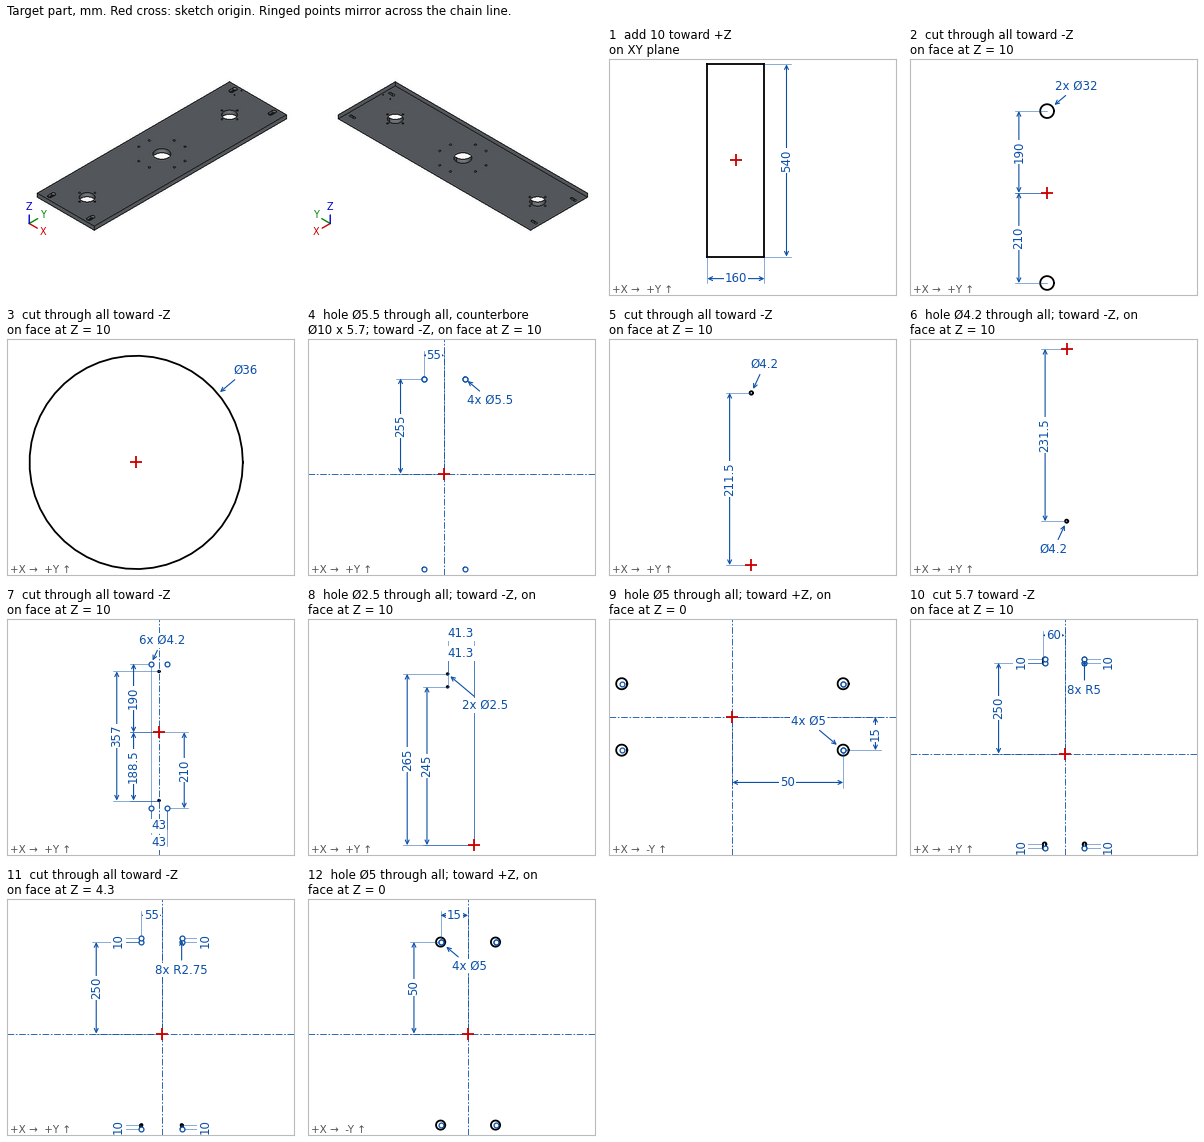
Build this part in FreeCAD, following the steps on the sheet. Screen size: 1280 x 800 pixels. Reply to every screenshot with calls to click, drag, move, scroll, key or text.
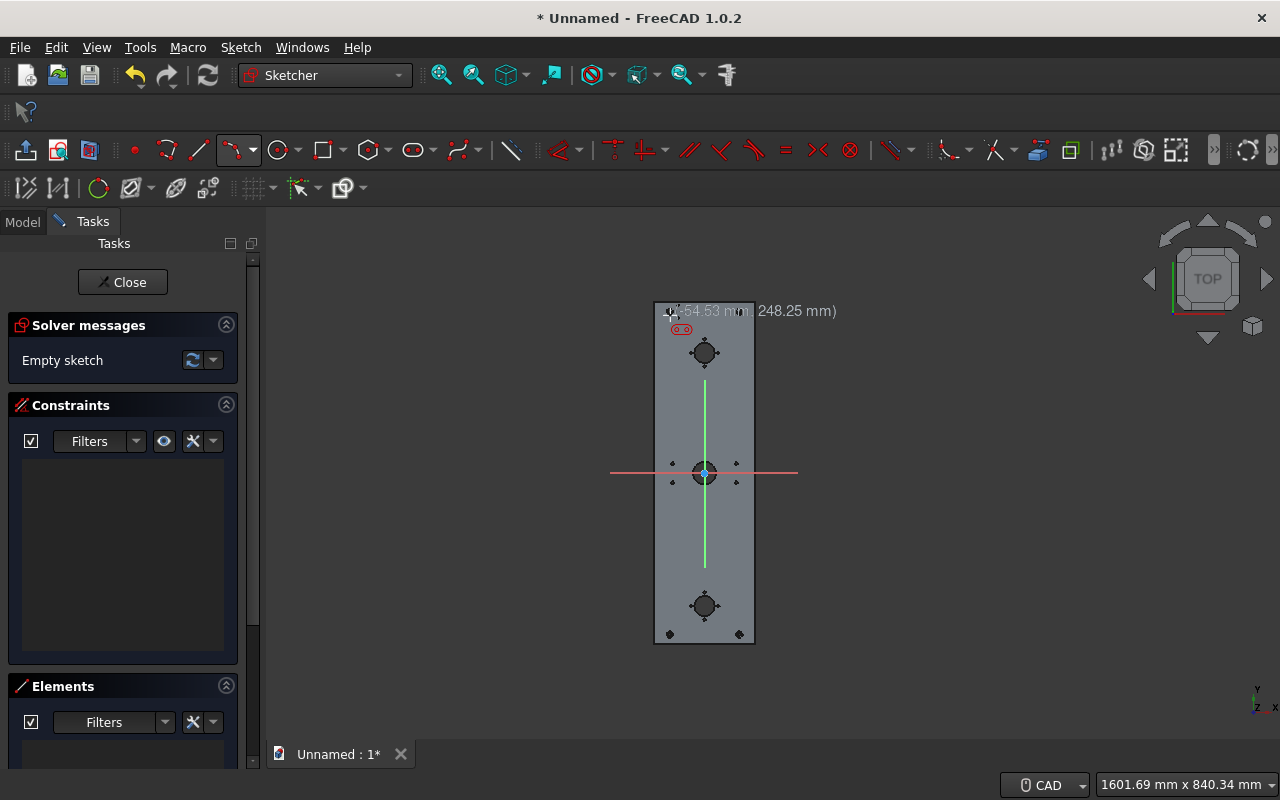
click(670, 315)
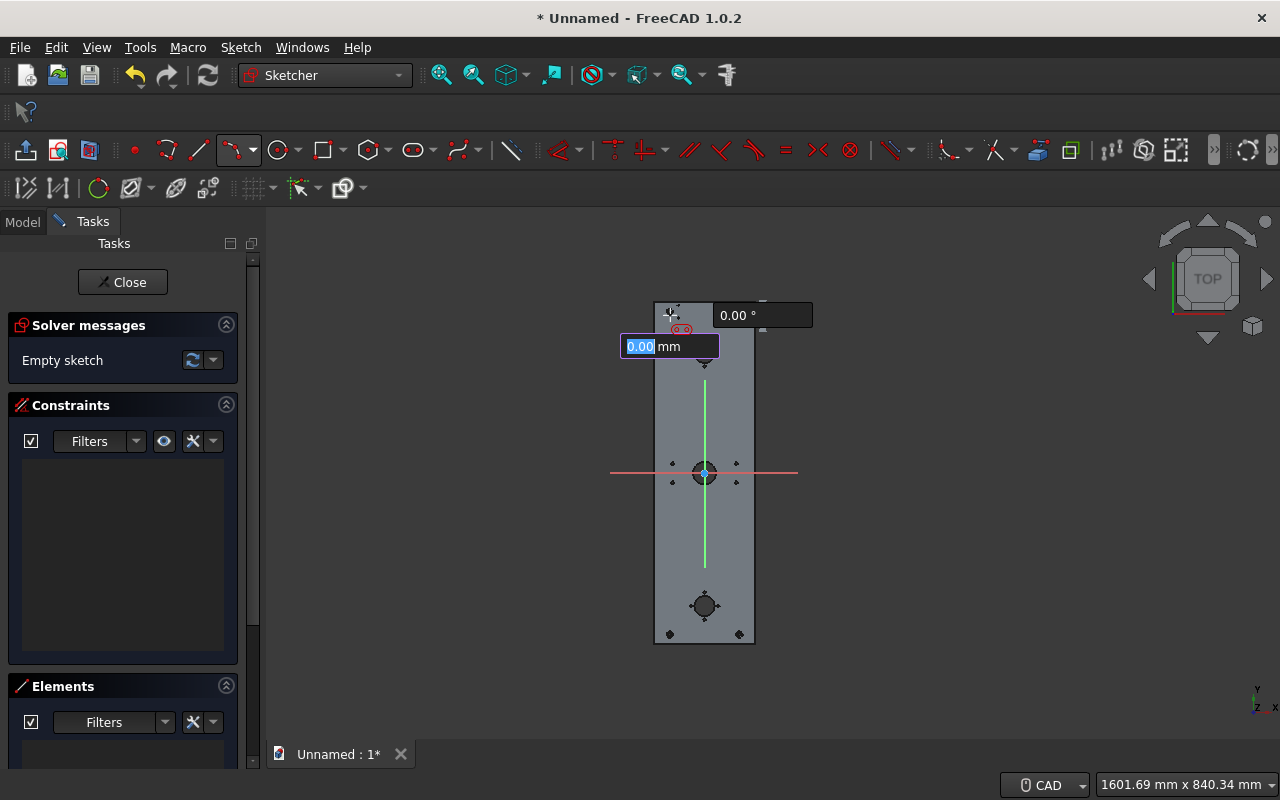
scroll(670, 309, up, 5)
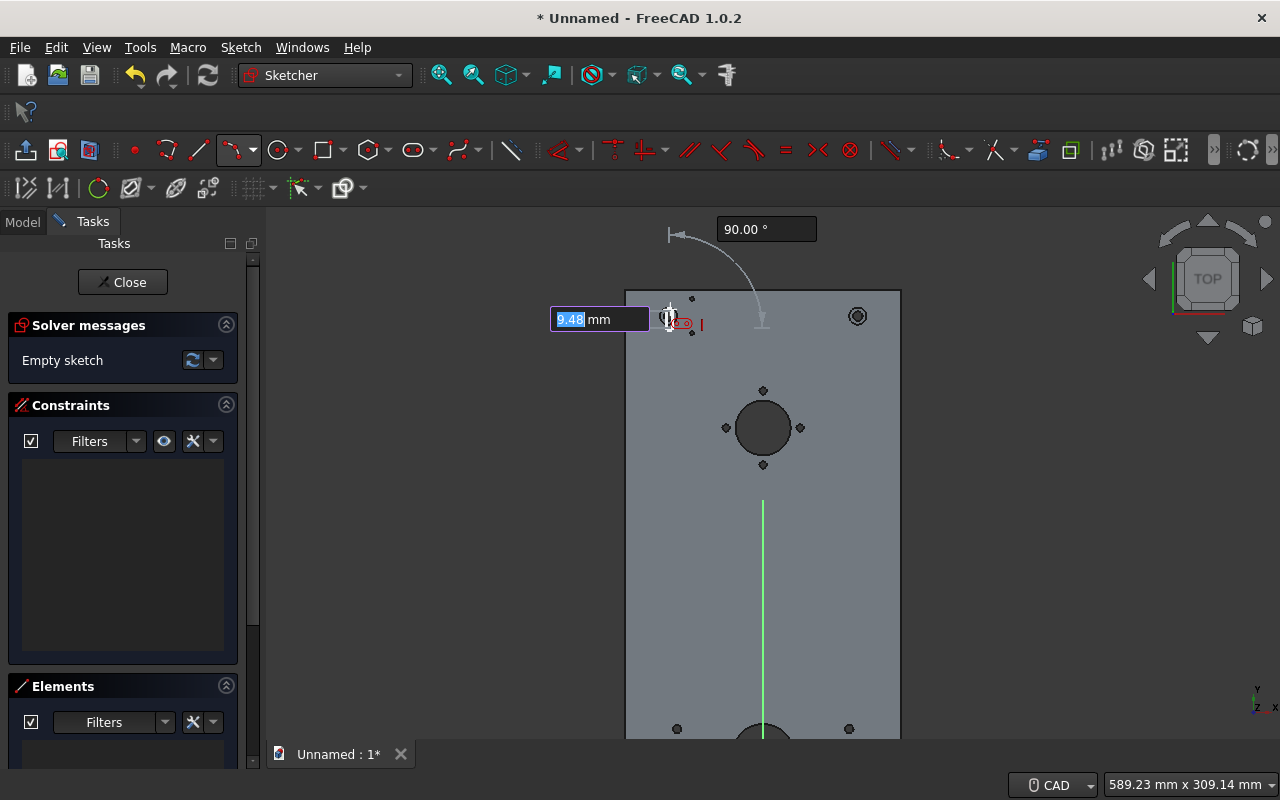
click(669, 307)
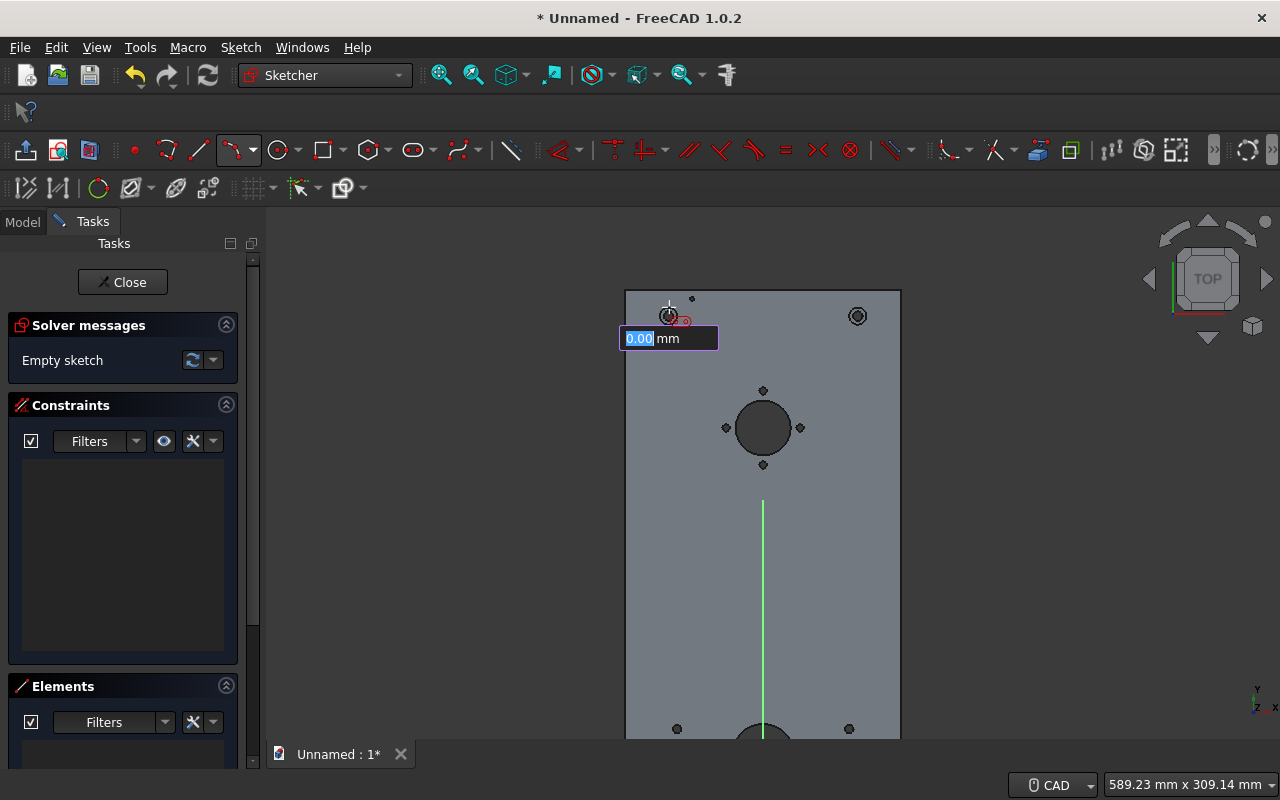
scroll(677, 316, up, 4)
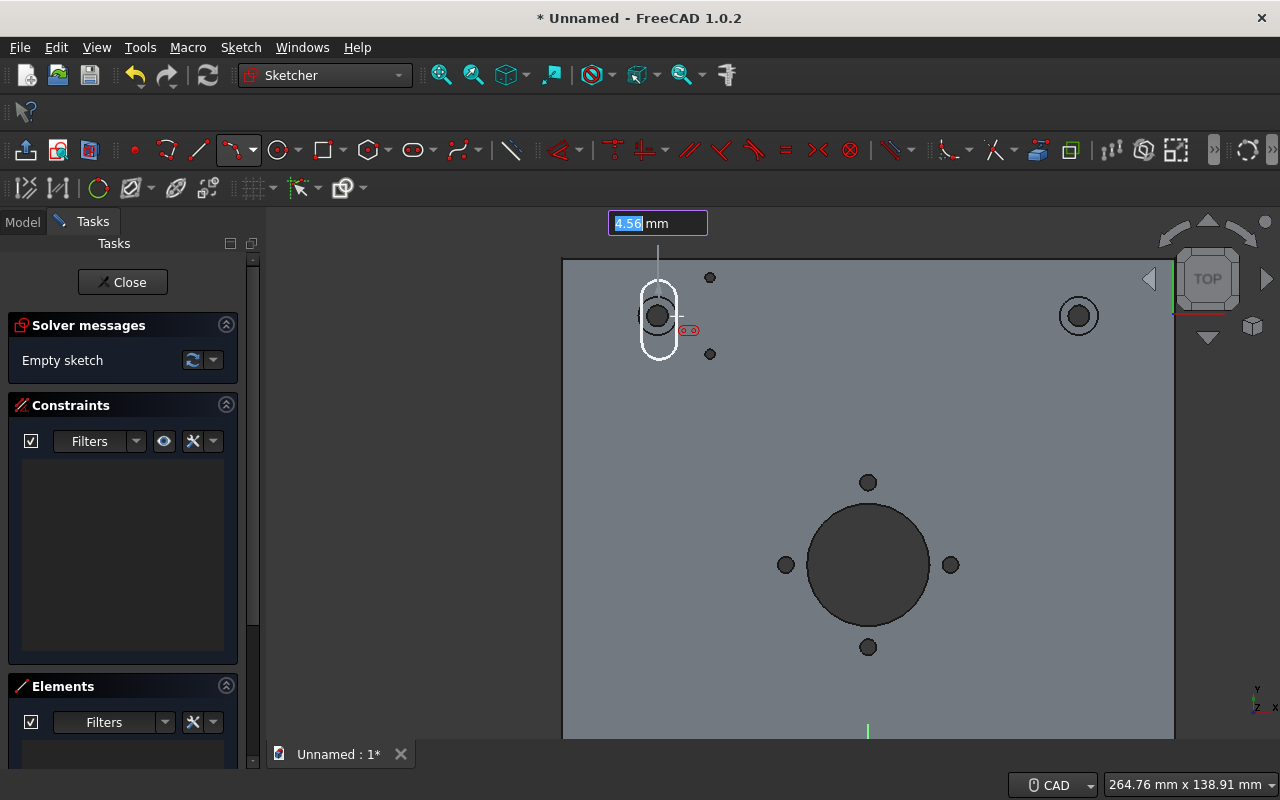
click(677, 316)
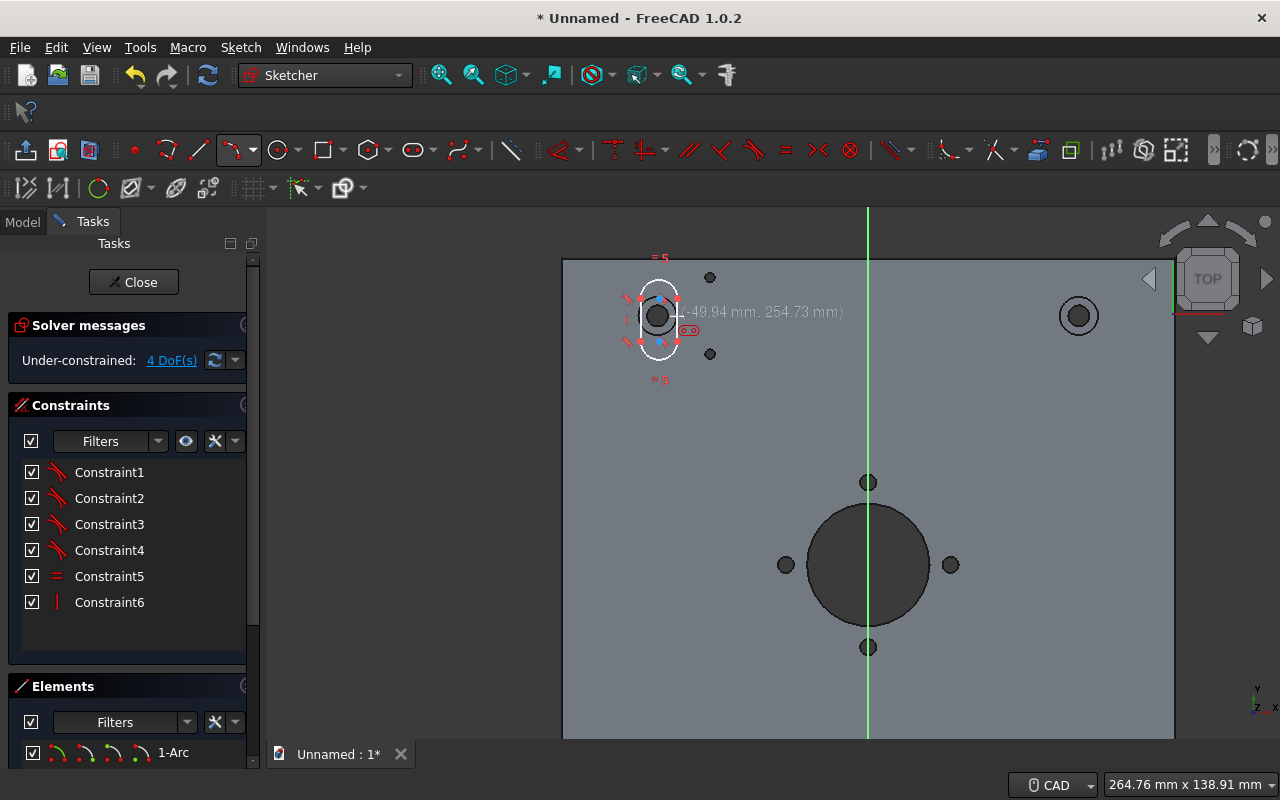
scroll(672, 311, down, 9)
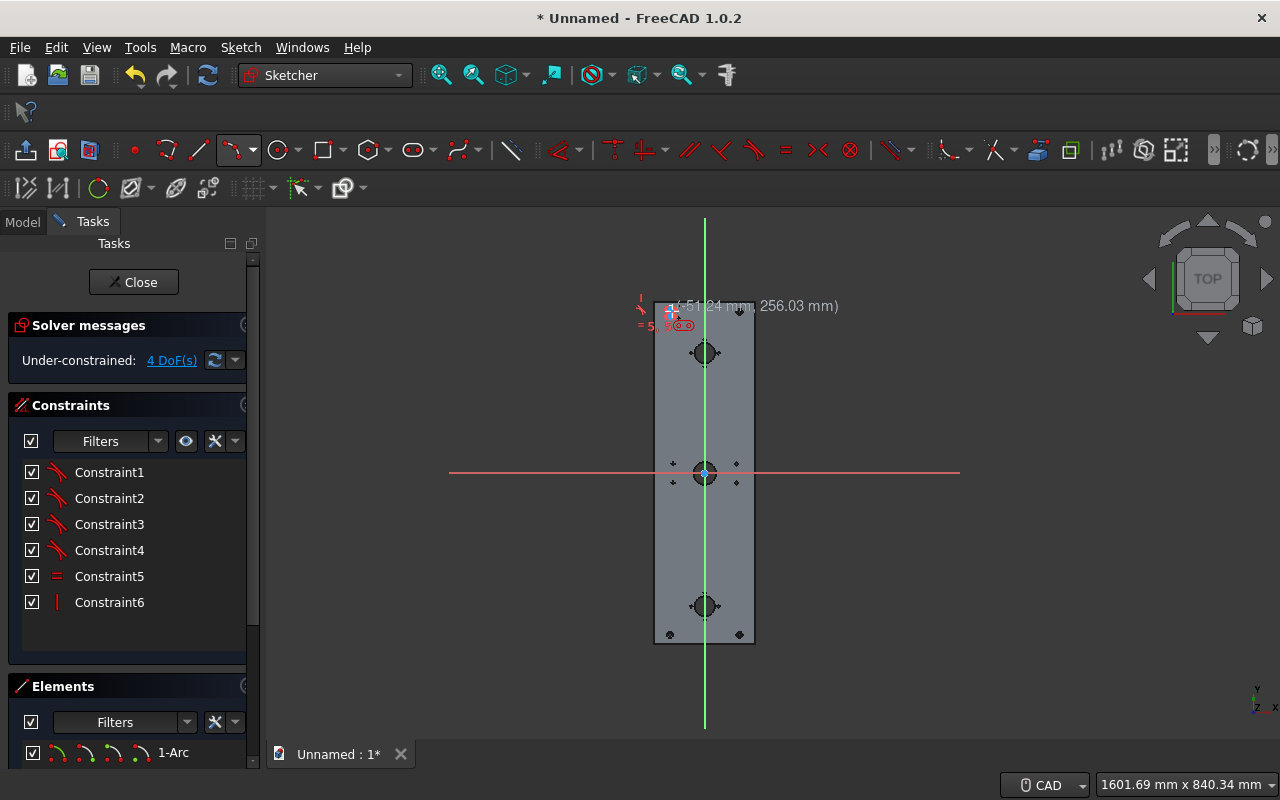
click(740, 315)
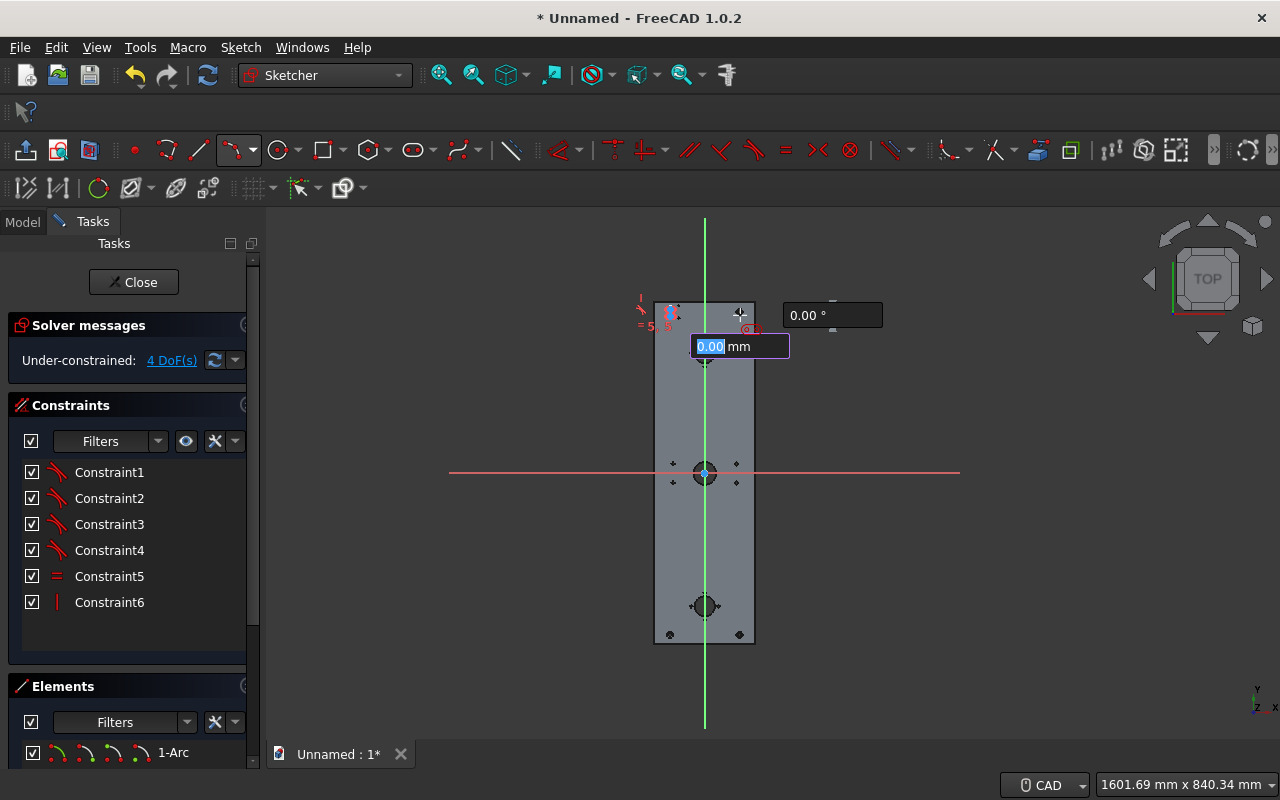
scroll(740, 309, up, 5)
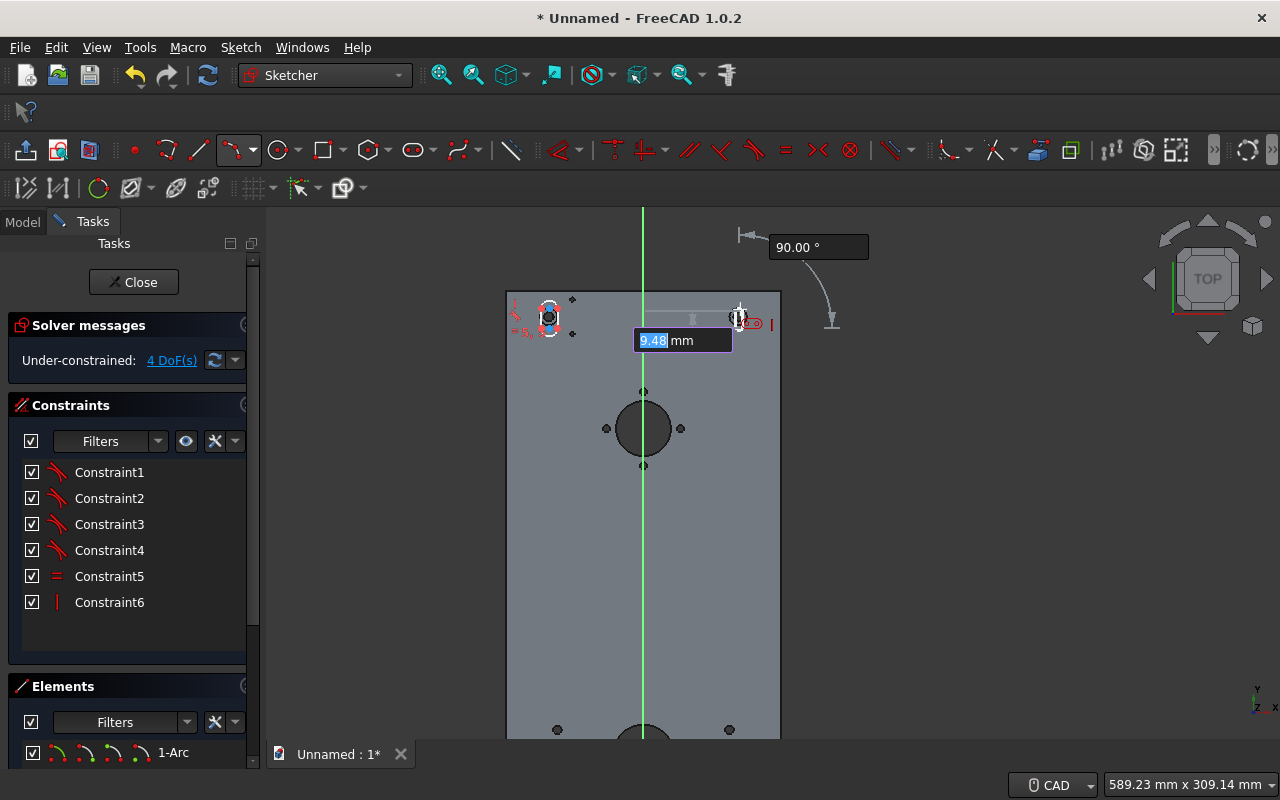
click(739, 308)